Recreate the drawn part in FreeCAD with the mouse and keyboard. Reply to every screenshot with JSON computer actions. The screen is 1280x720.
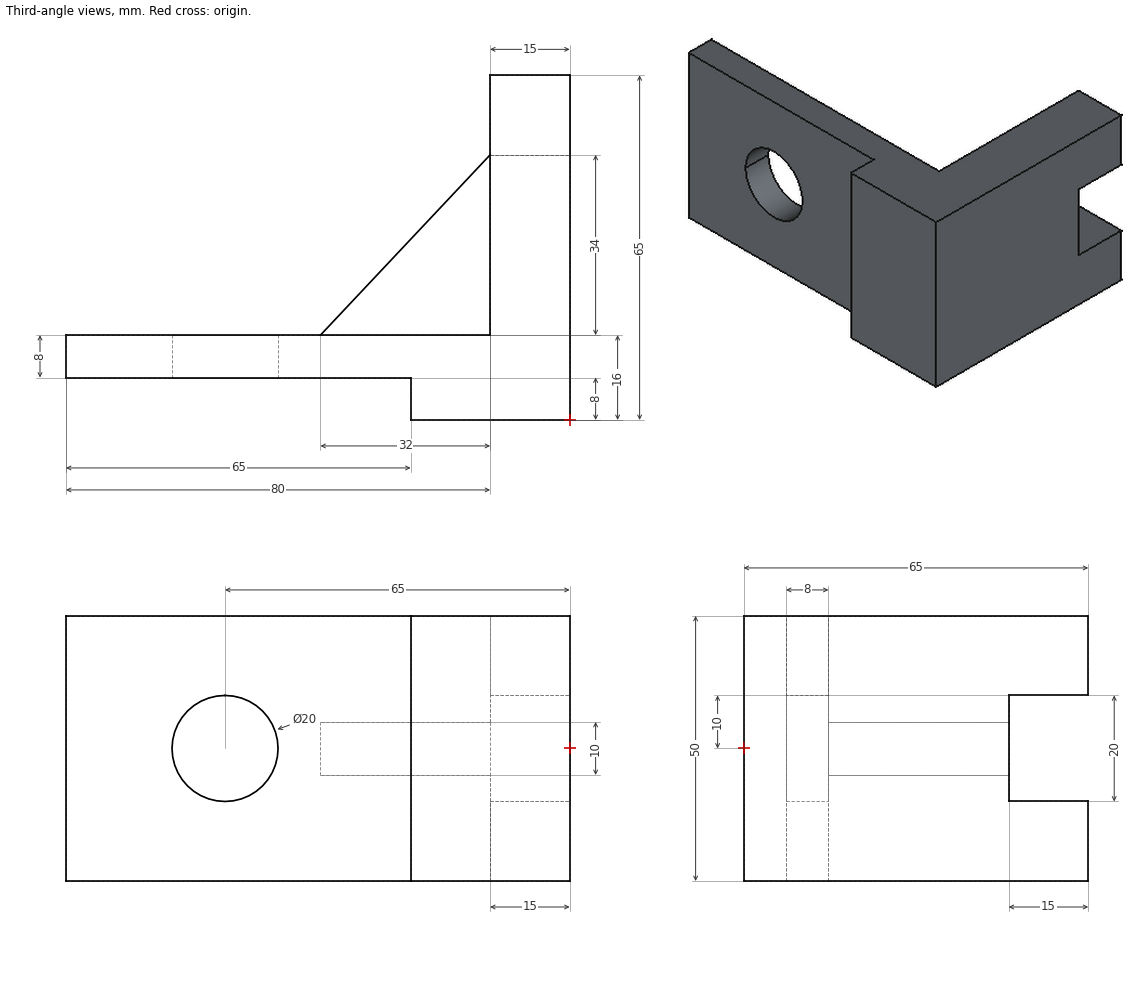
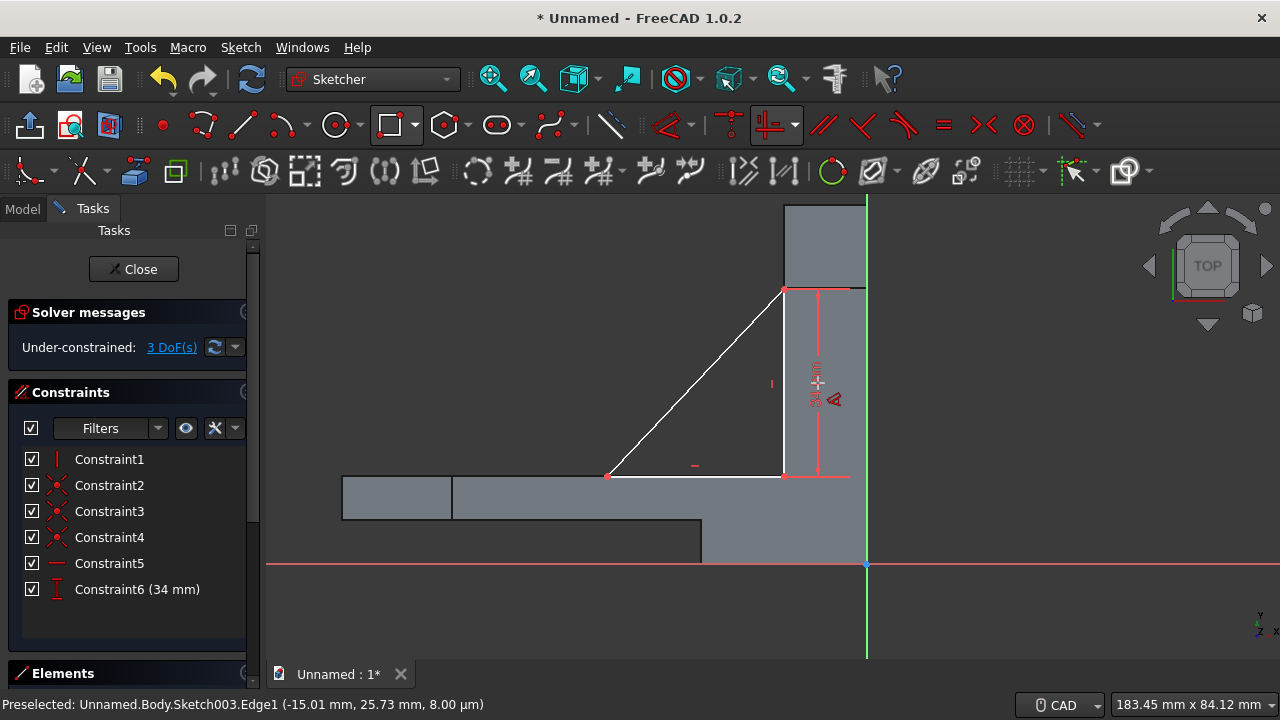
{"action": "left_click", "coordinate": [660, 477]}
{"action": "left_click", "coordinate": [695, 511]}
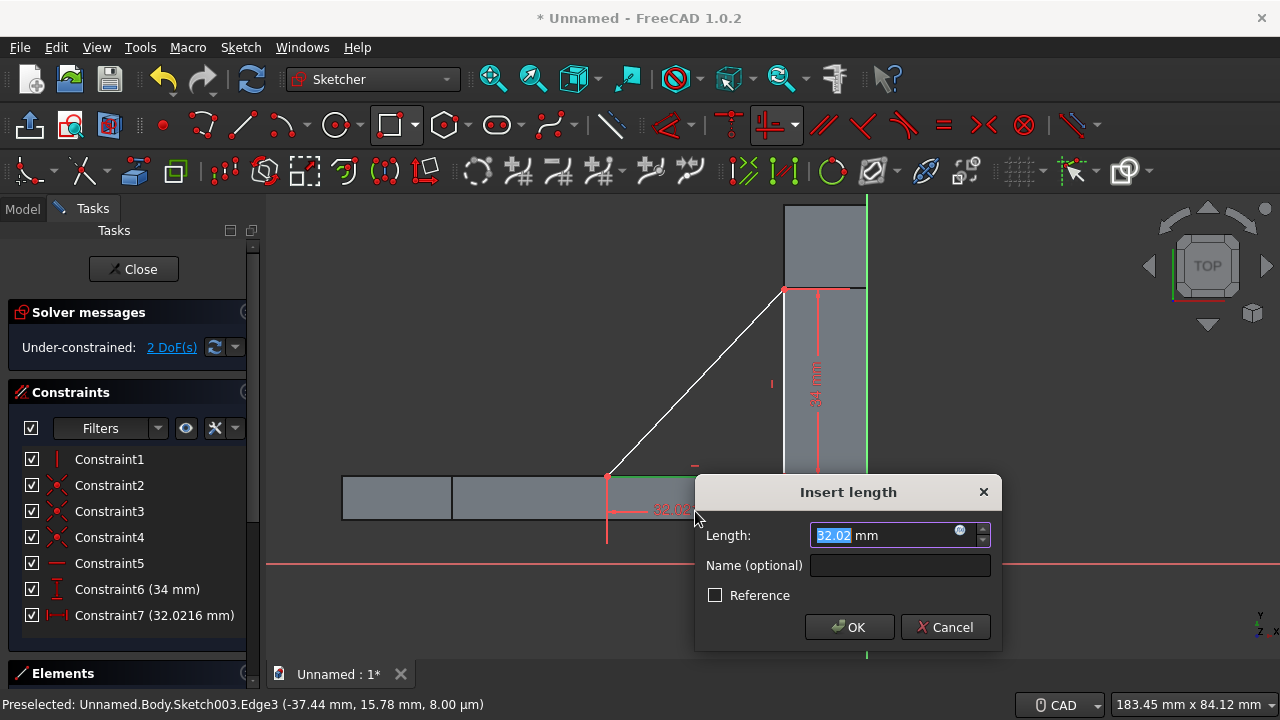
{"action": "type", "text": "32"}
{"action": "key", "text": "Return"}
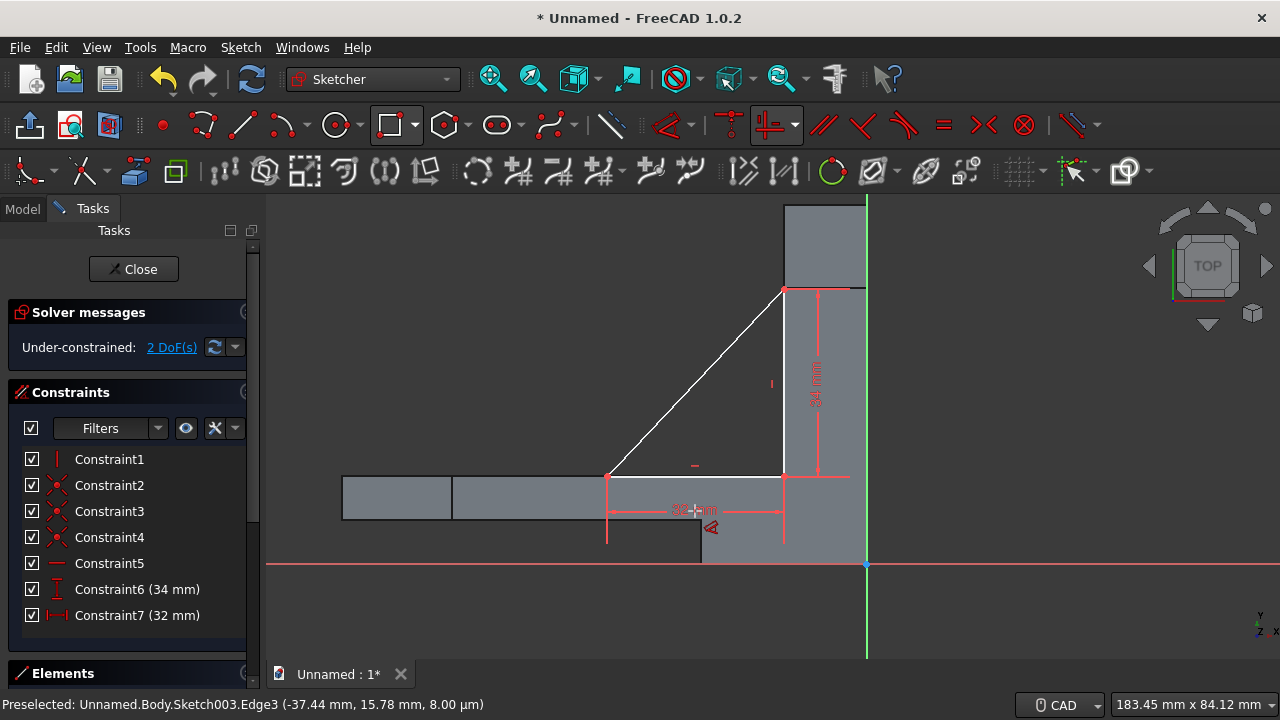
{"action": "left_click", "coordinate": [784, 477]}
{"action": "left_click", "coordinate": [825, 598]}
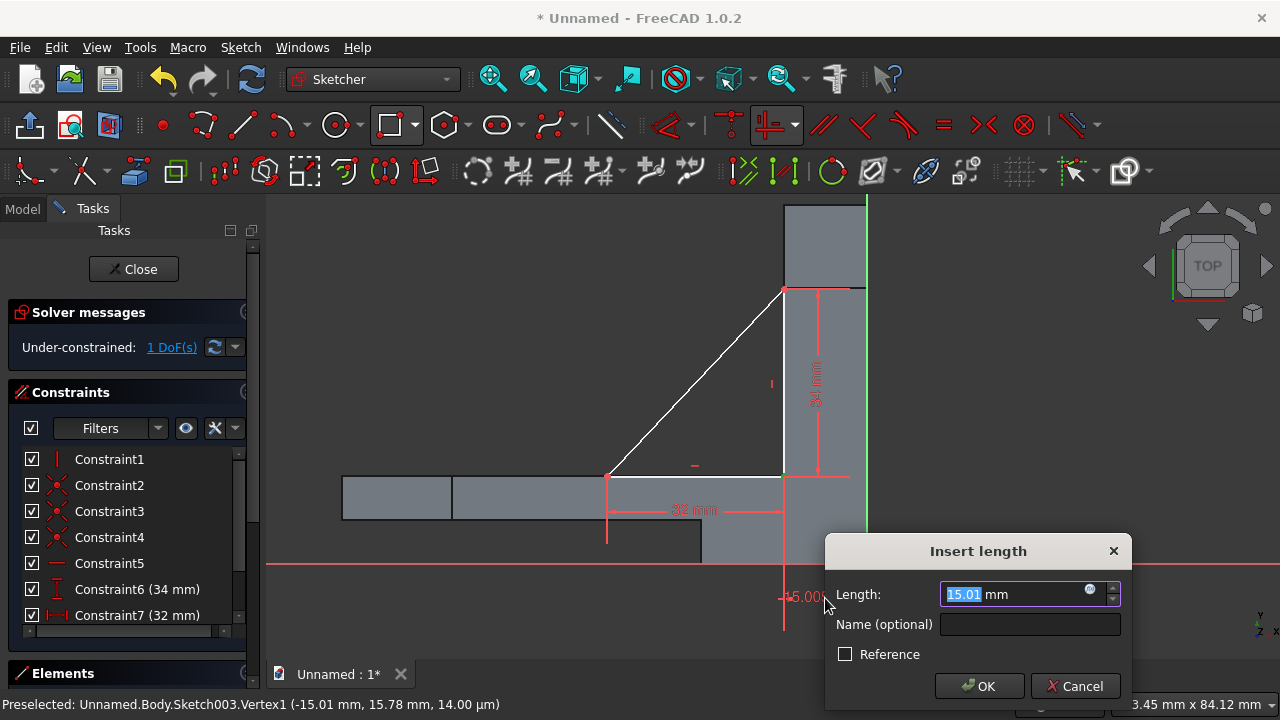
{"action": "type", "text": "15"}
{"action": "key", "text": "Return"}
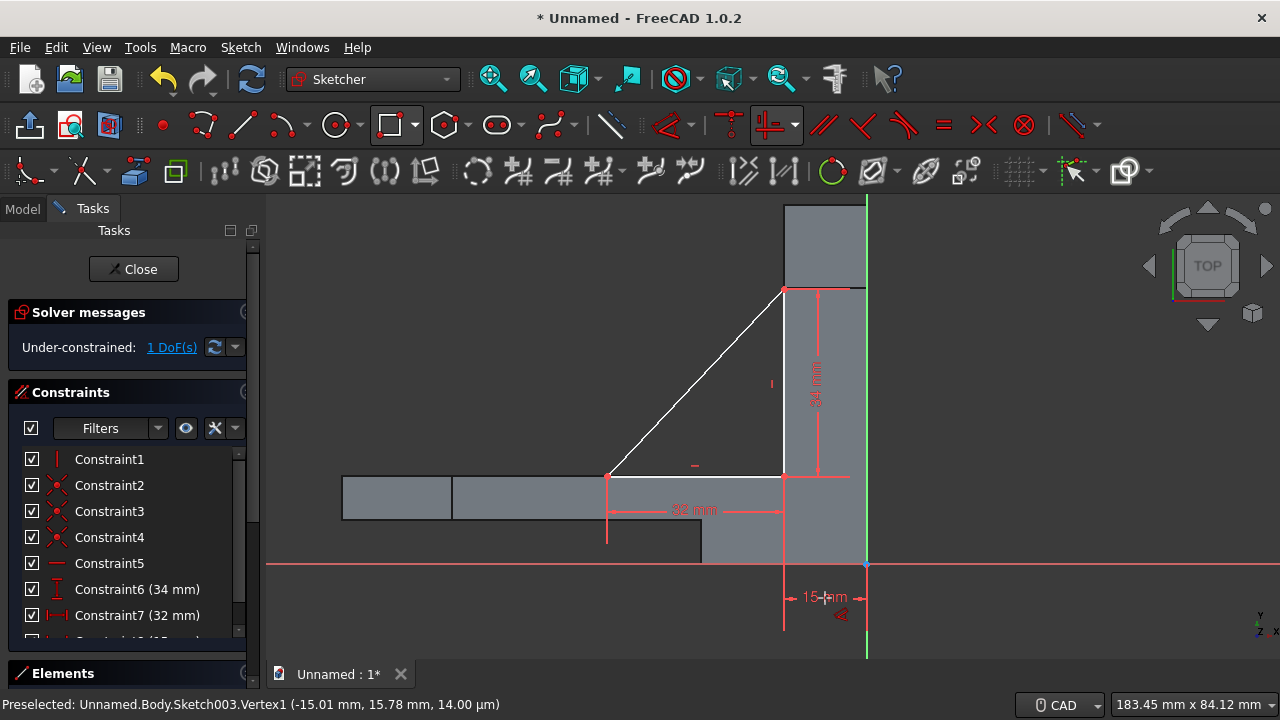
{"action": "left_click", "coordinate": [784, 477]}
{"action": "left_click", "coordinate": [901, 521]}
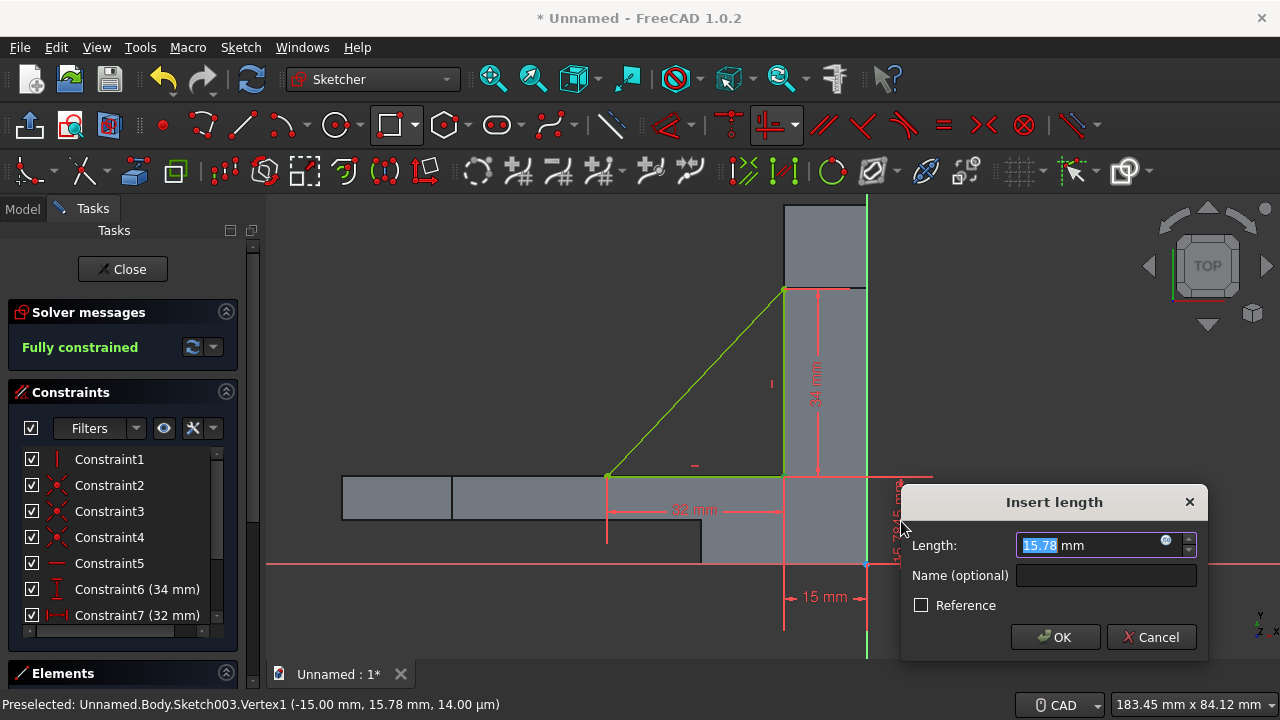
{"action": "type", "text": "16"}
{"action": "key", "text": "Return"}
{"action": "key", "text": "Escape"}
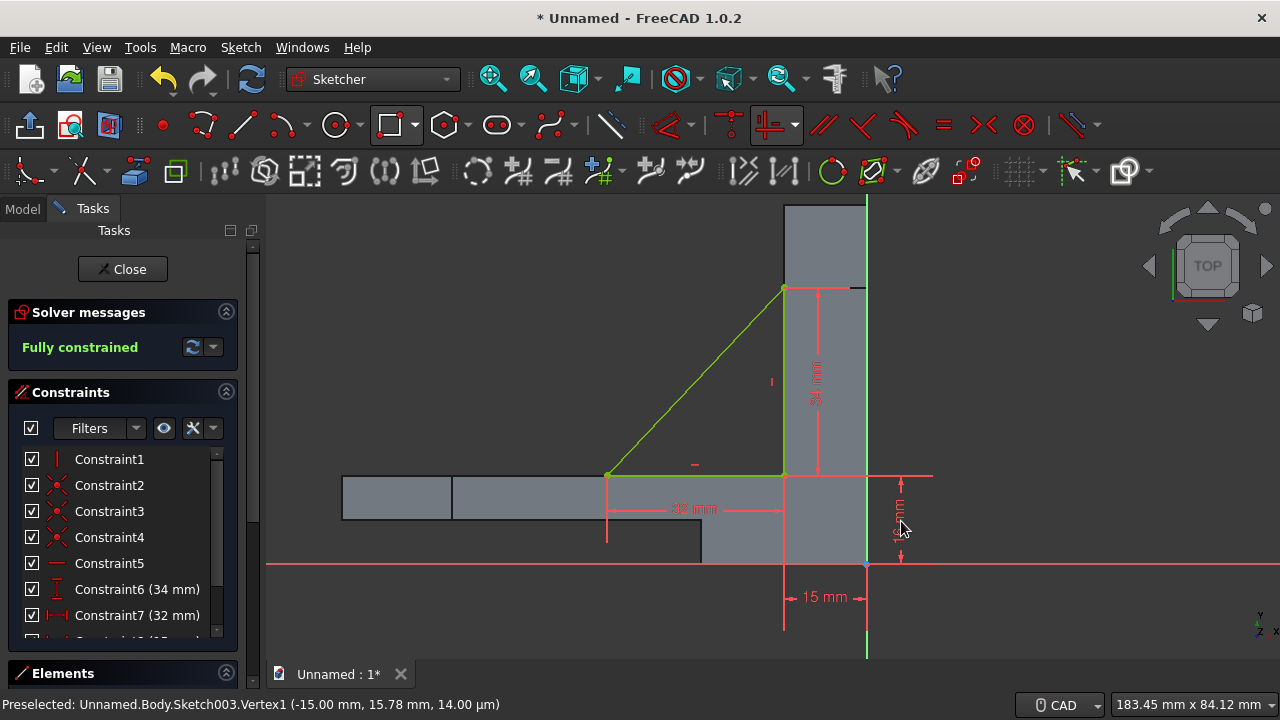
{"action": "left_click", "coordinate": [123, 269]}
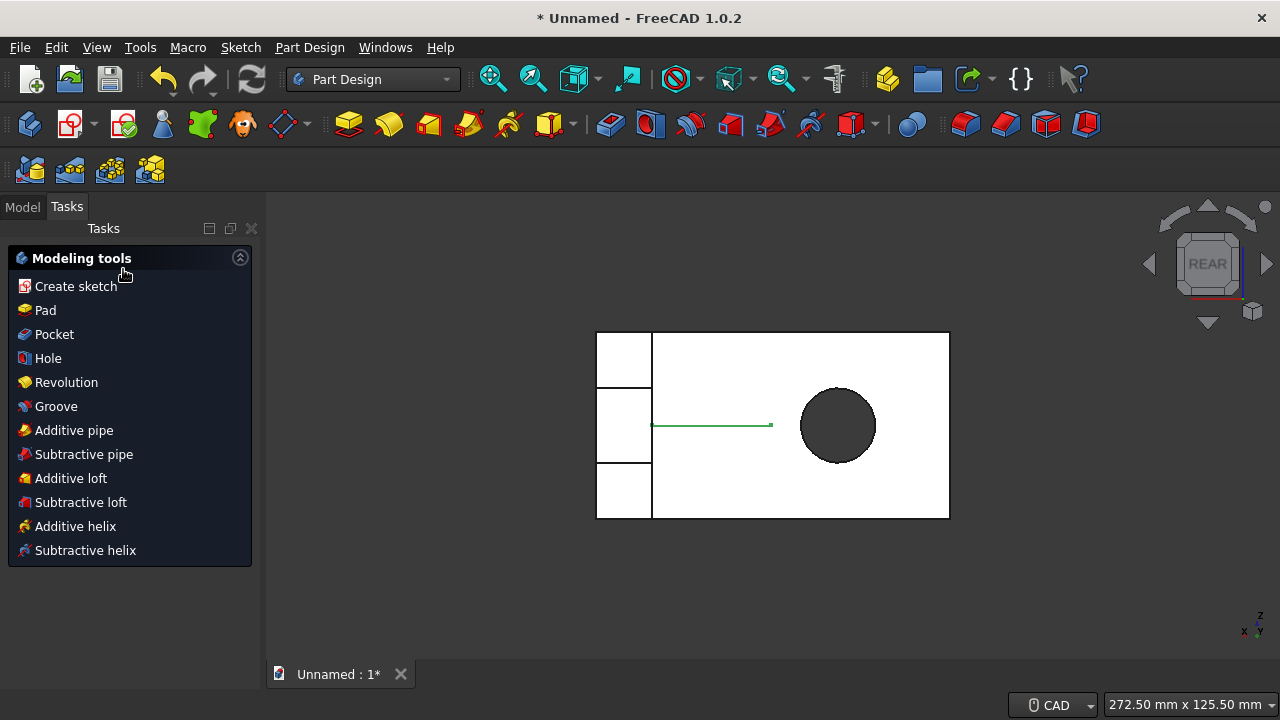
{"action": "left_click", "coordinate": [350, 124]}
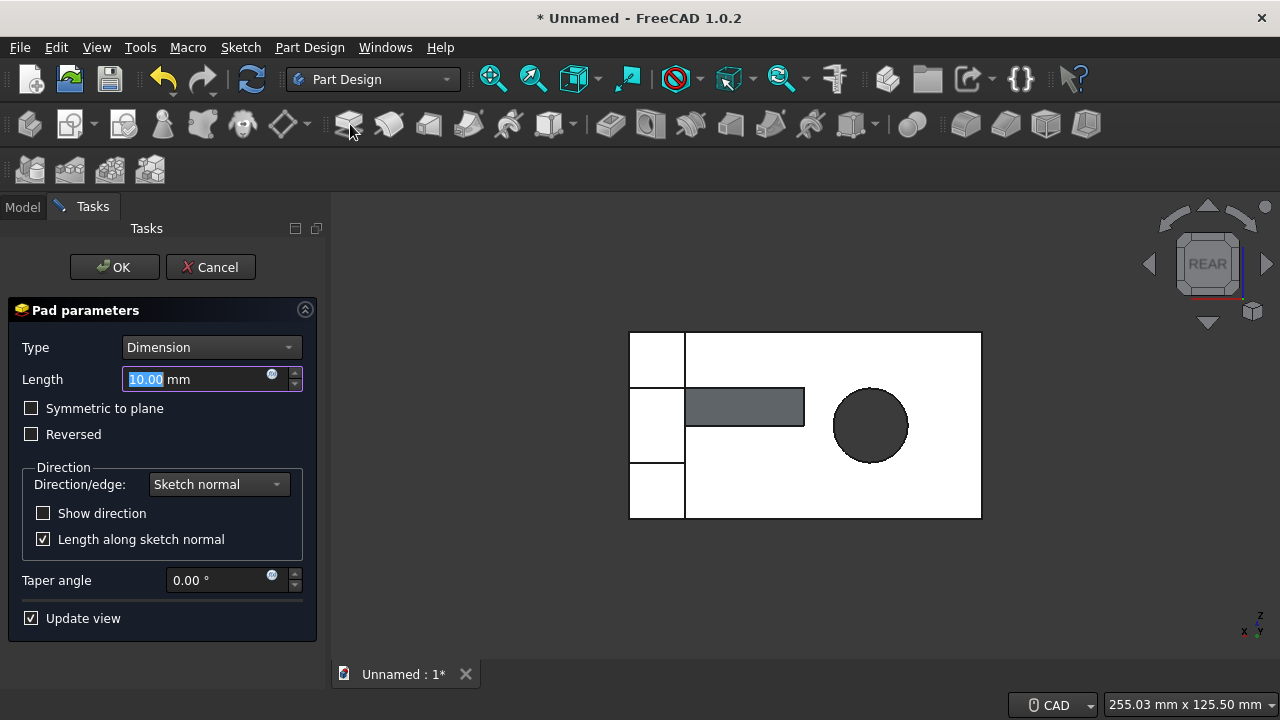
{"action": "type", "text": "10"}
{"action": "key", "text": "Tab"}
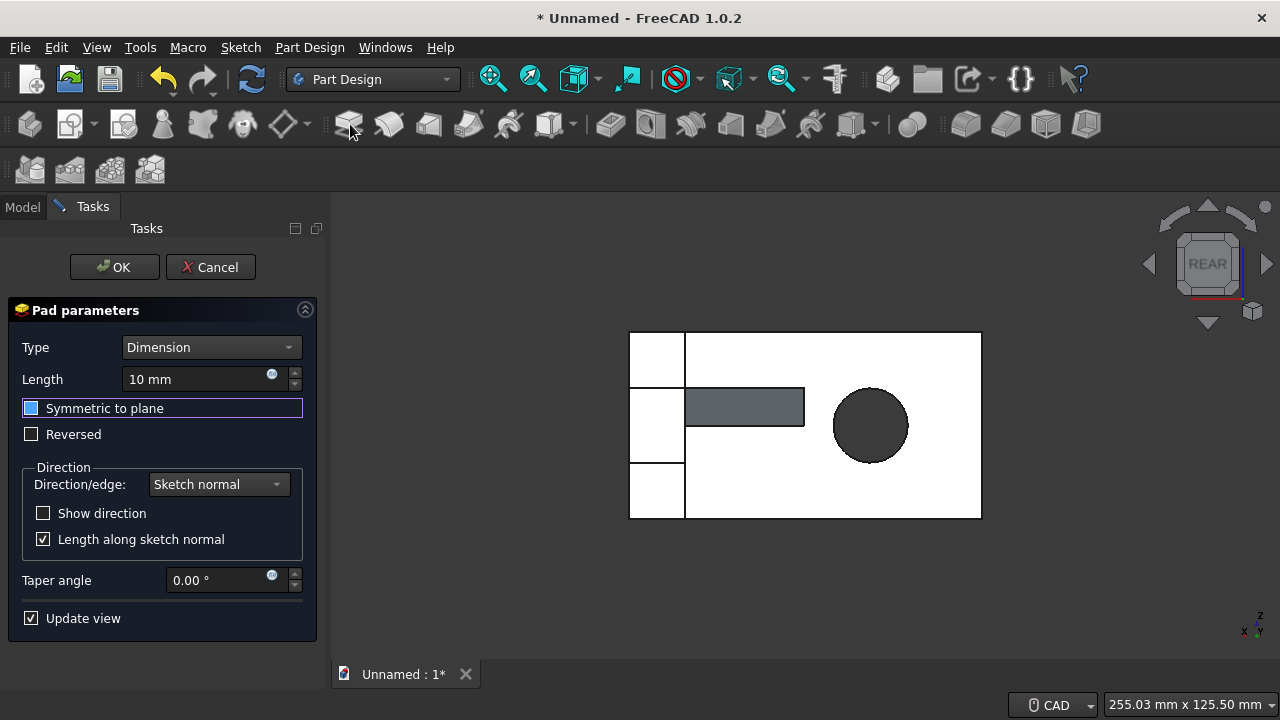
{"action": "left_click", "coordinate": [30, 408]}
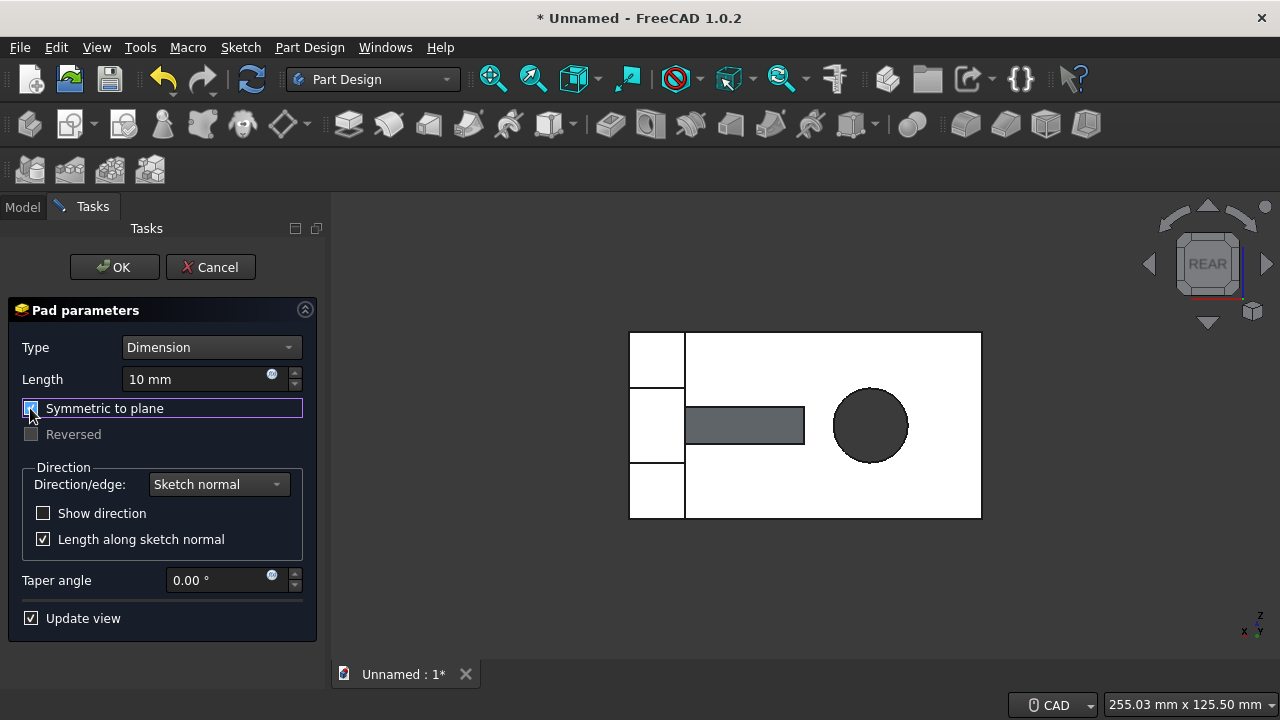
{"action": "left_click", "coordinate": [115, 267]}